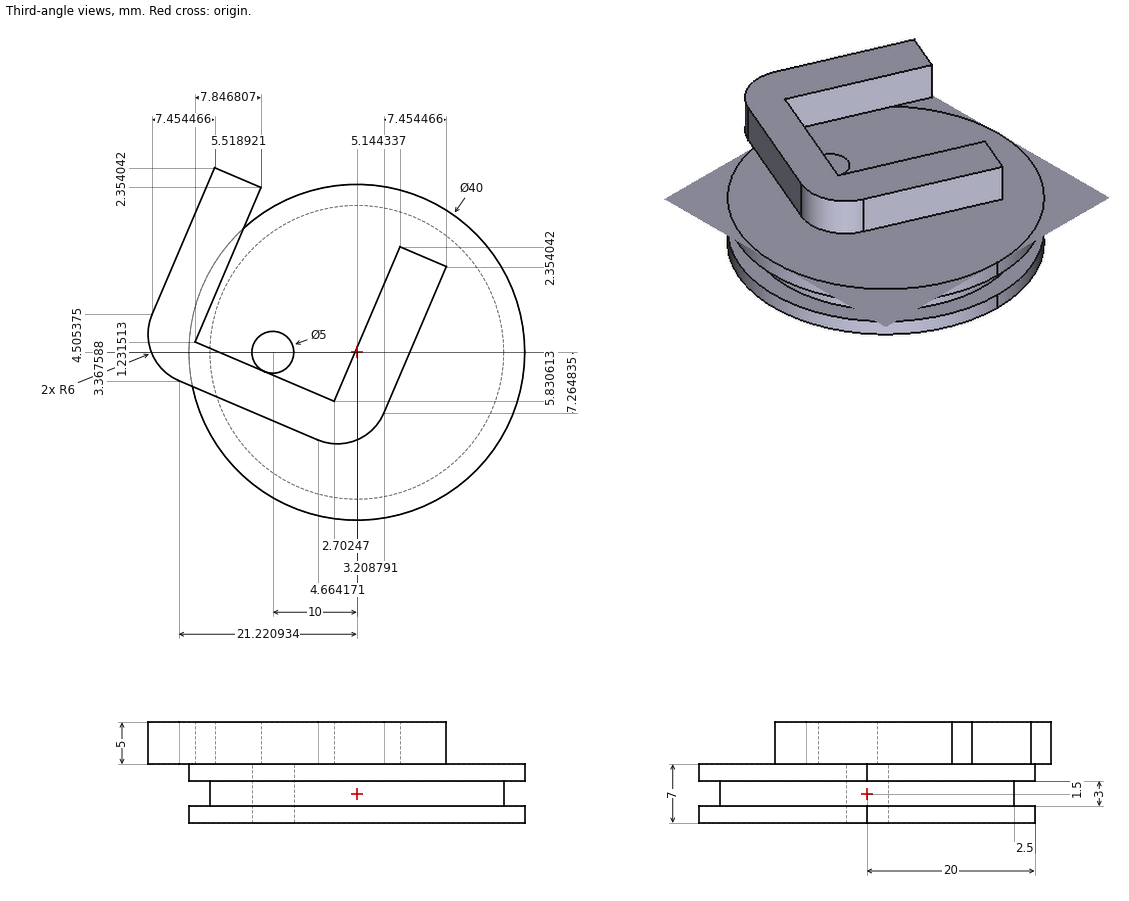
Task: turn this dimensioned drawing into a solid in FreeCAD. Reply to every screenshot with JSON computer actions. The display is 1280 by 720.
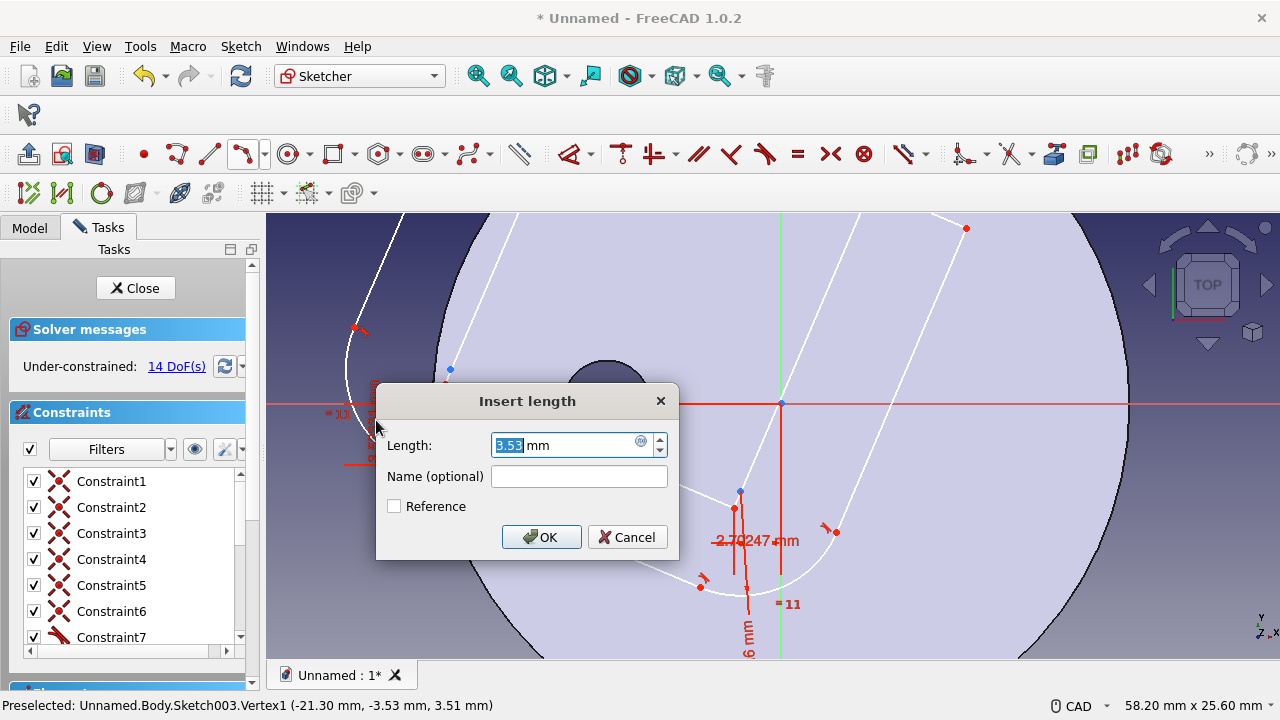
{"action": "type", "text": "3.367588"}
{"action": "key", "text": "Return"}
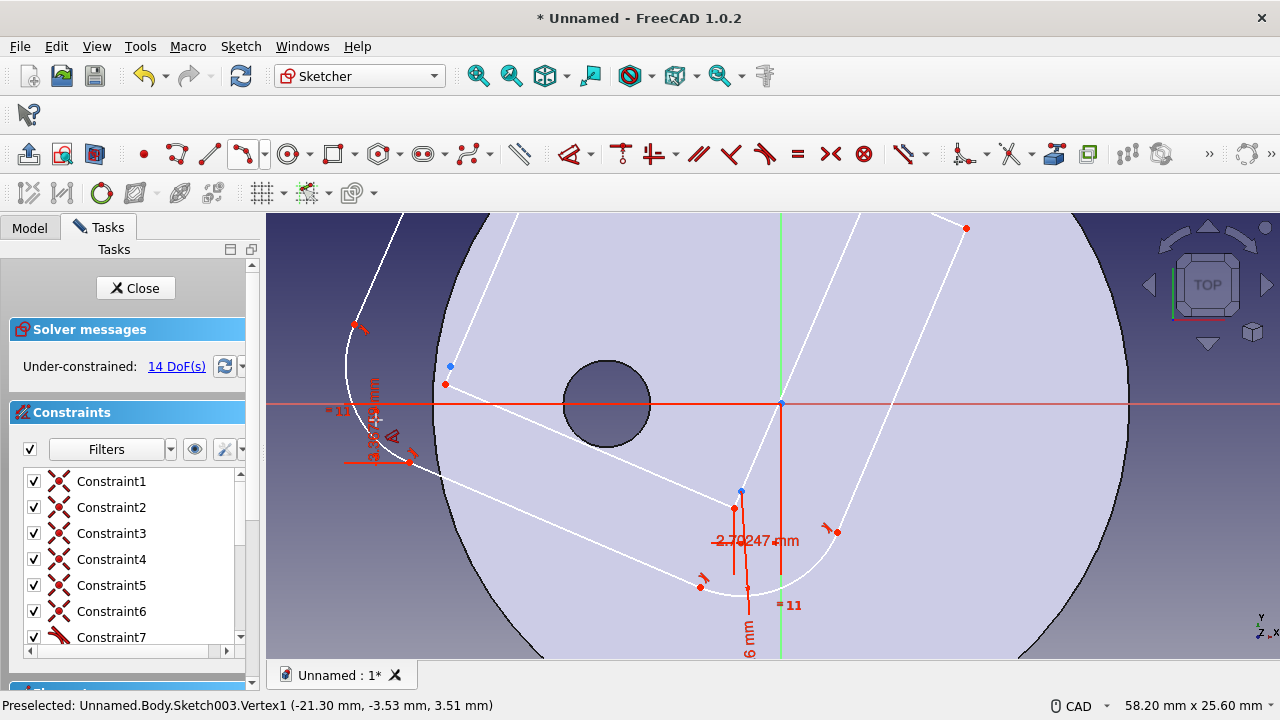
{"action": "left_click", "coordinate": [700, 588]}
{"action": "left_click", "coordinate": [741, 622]}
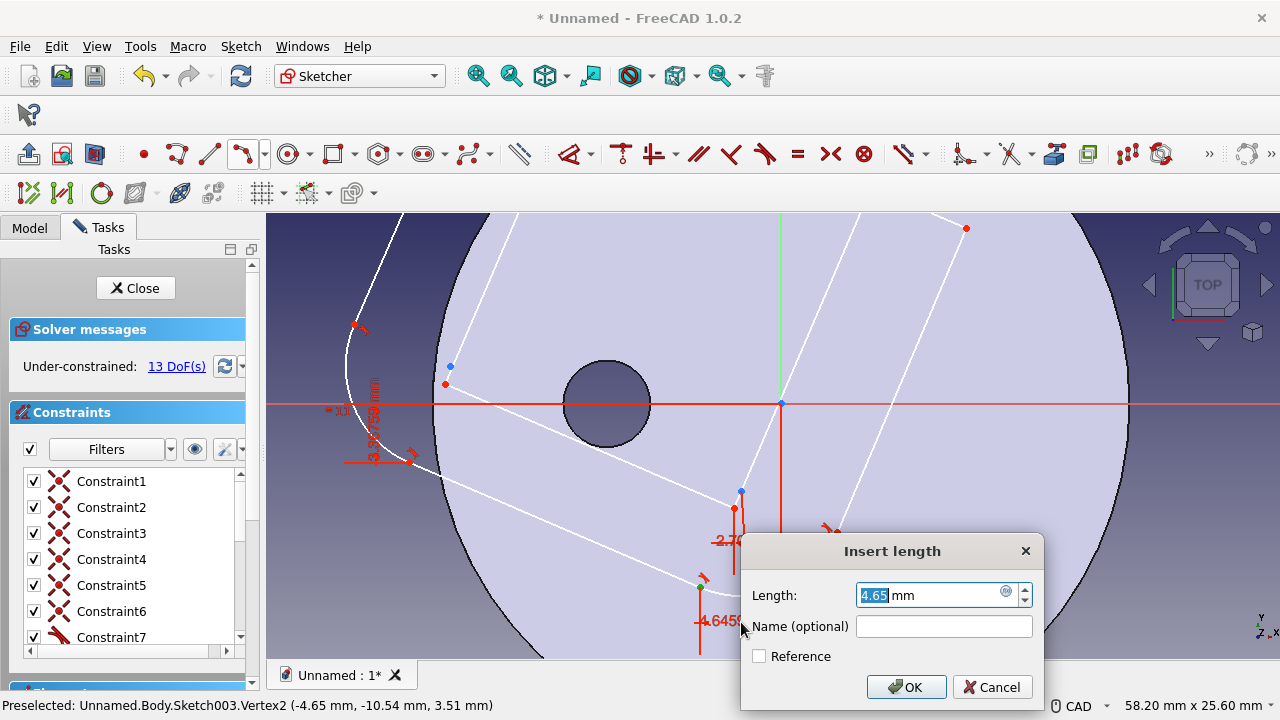
{"action": "type", "text": "4.664171"}
{"action": "key", "text": "Return"}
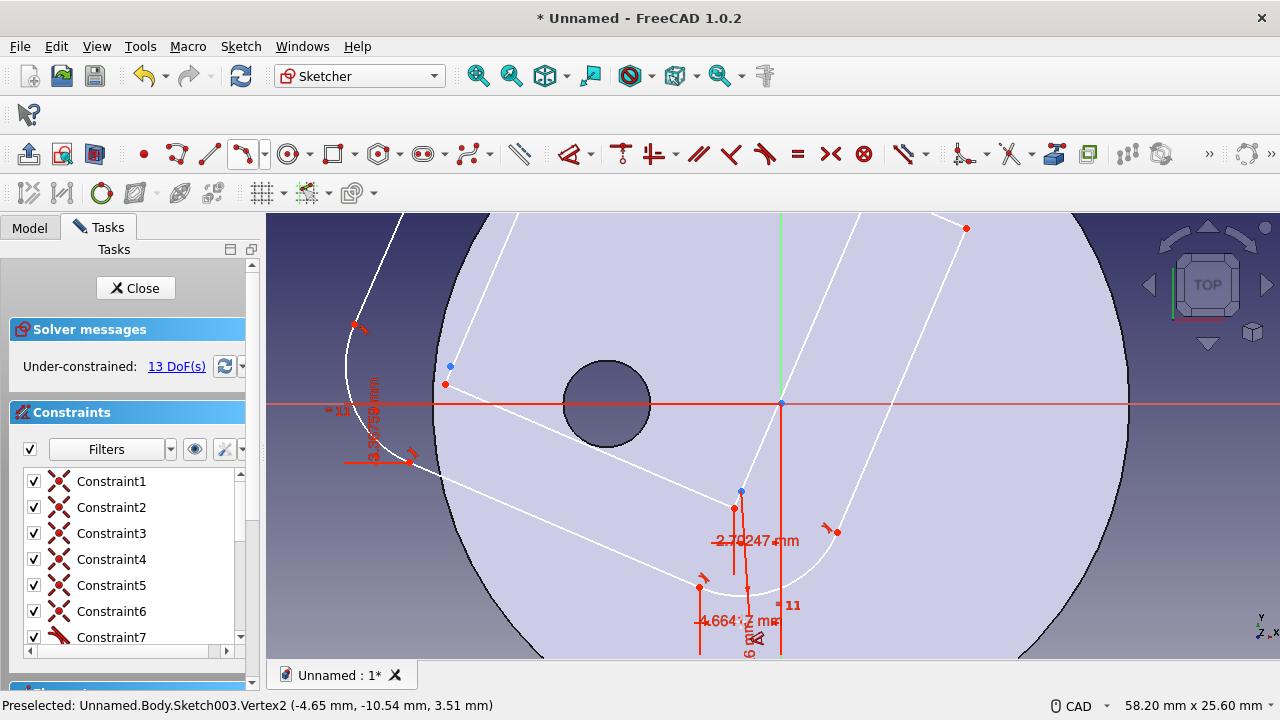
{"action": "left_click", "coordinate": [837, 532]}
{"action": "left_click", "coordinate": [809, 370]}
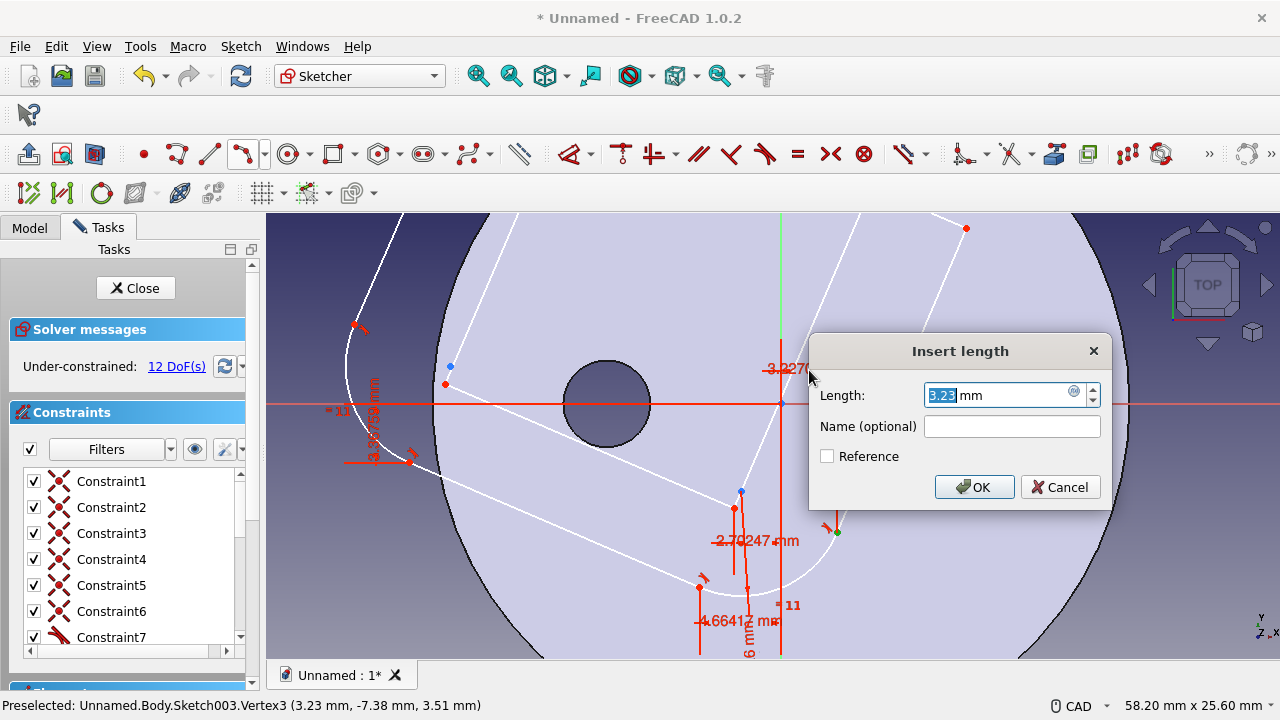
{"action": "type", "text": "3.208791"}
{"action": "key", "text": "Return"}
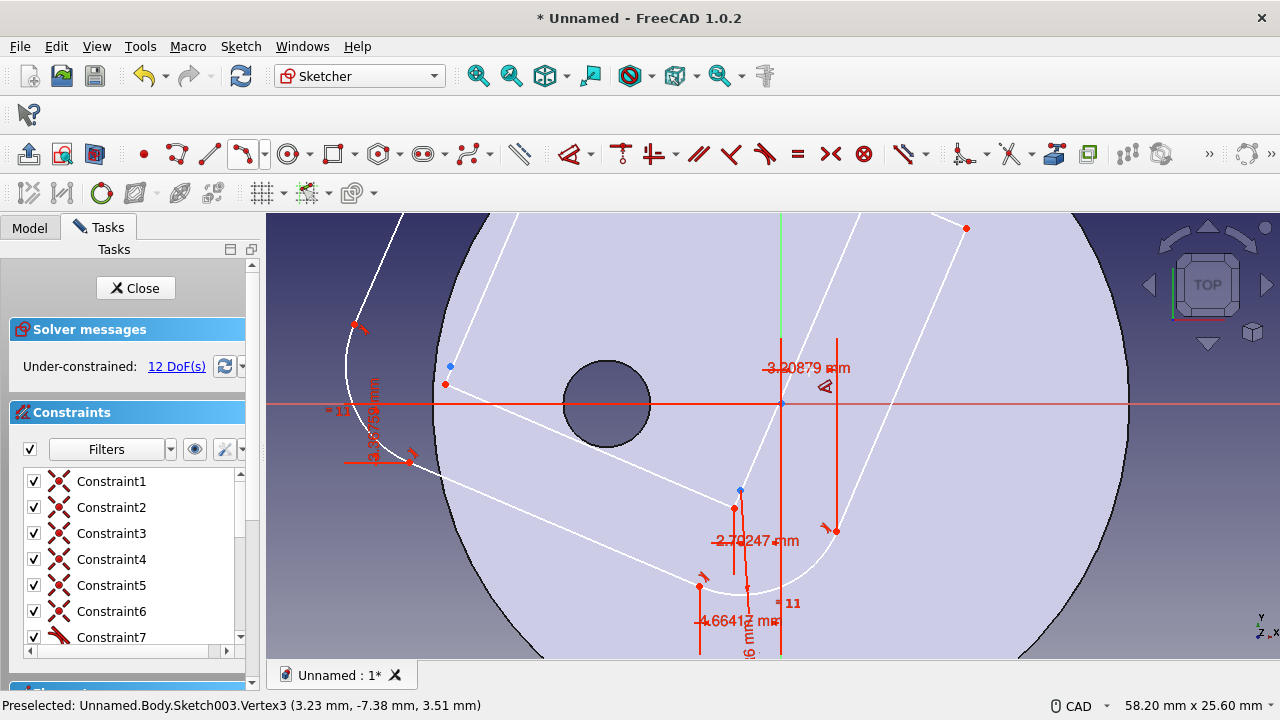
{"action": "left_click", "coordinate": [837, 531]}
{"action": "left_click", "coordinate": [871, 497]}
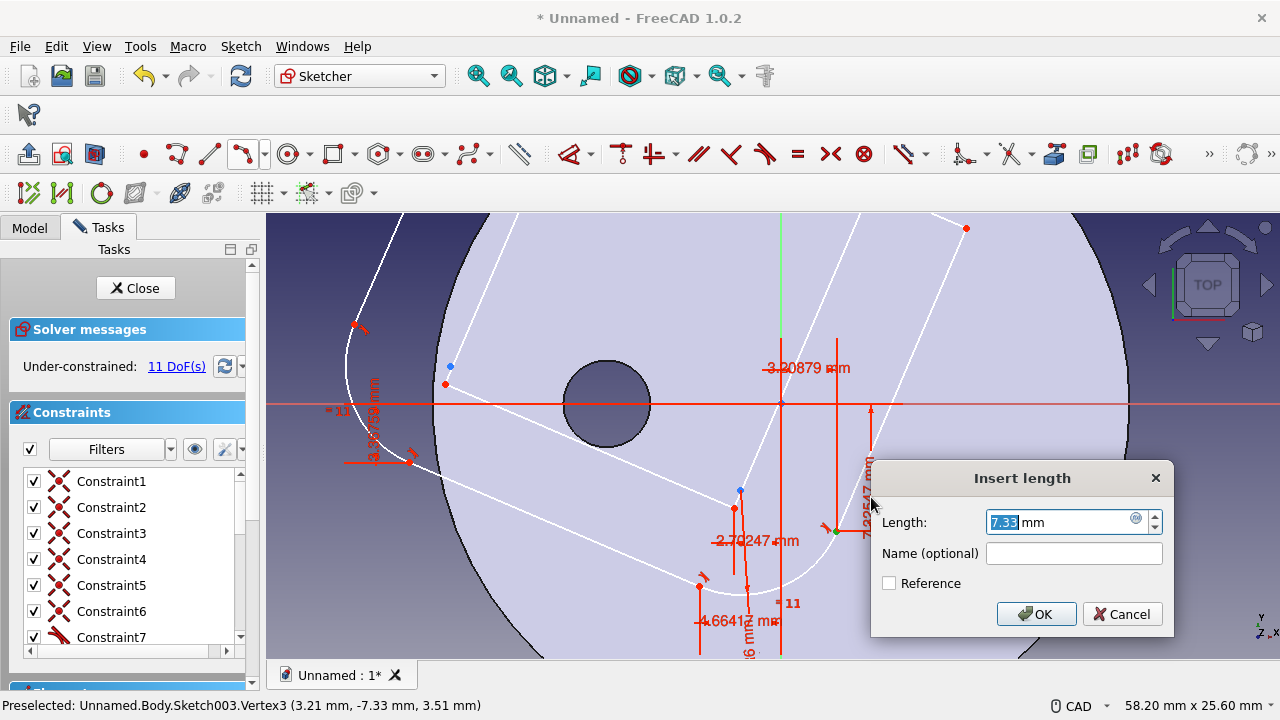
{"action": "type", "text": "7.264835"}
{"action": "key", "text": "Return"}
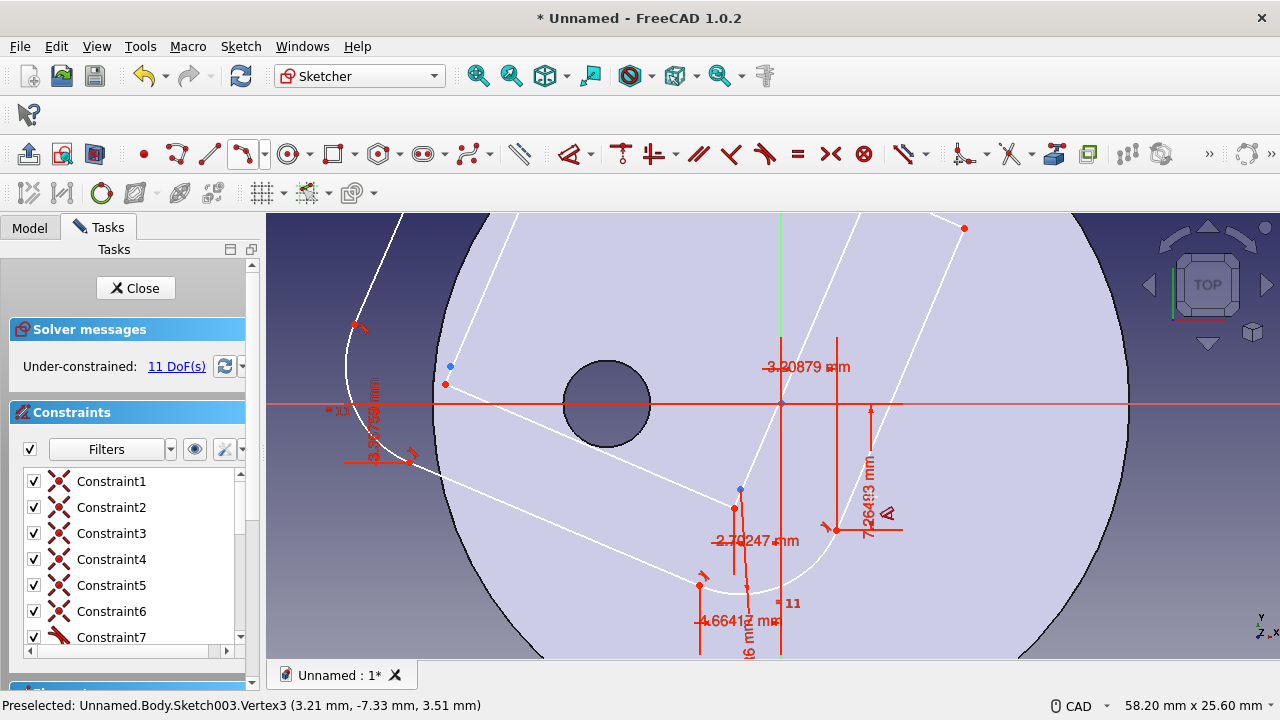
{"action": "scroll", "coordinate": [740, 544], "scroll_direction": "down", "scroll_amount": 4}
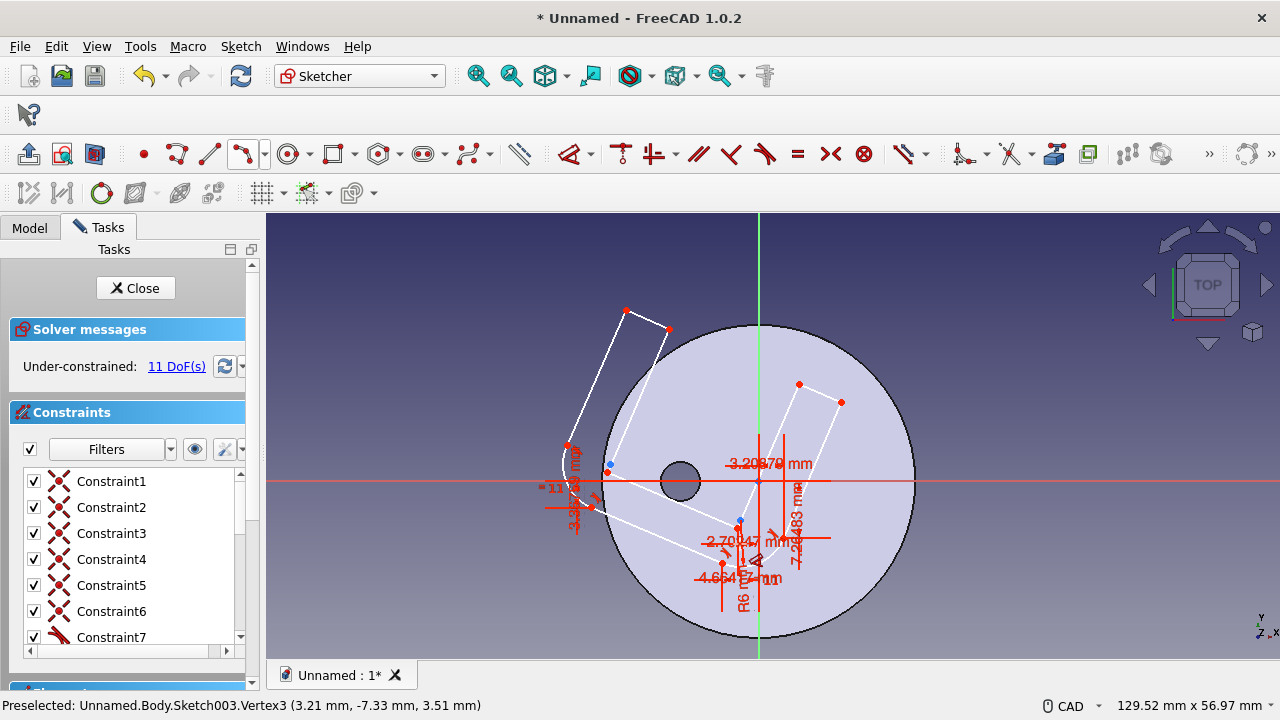
{"action": "left_click", "coordinate": [799, 384]}
{"action": "left_click", "coordinate": [779, 350]}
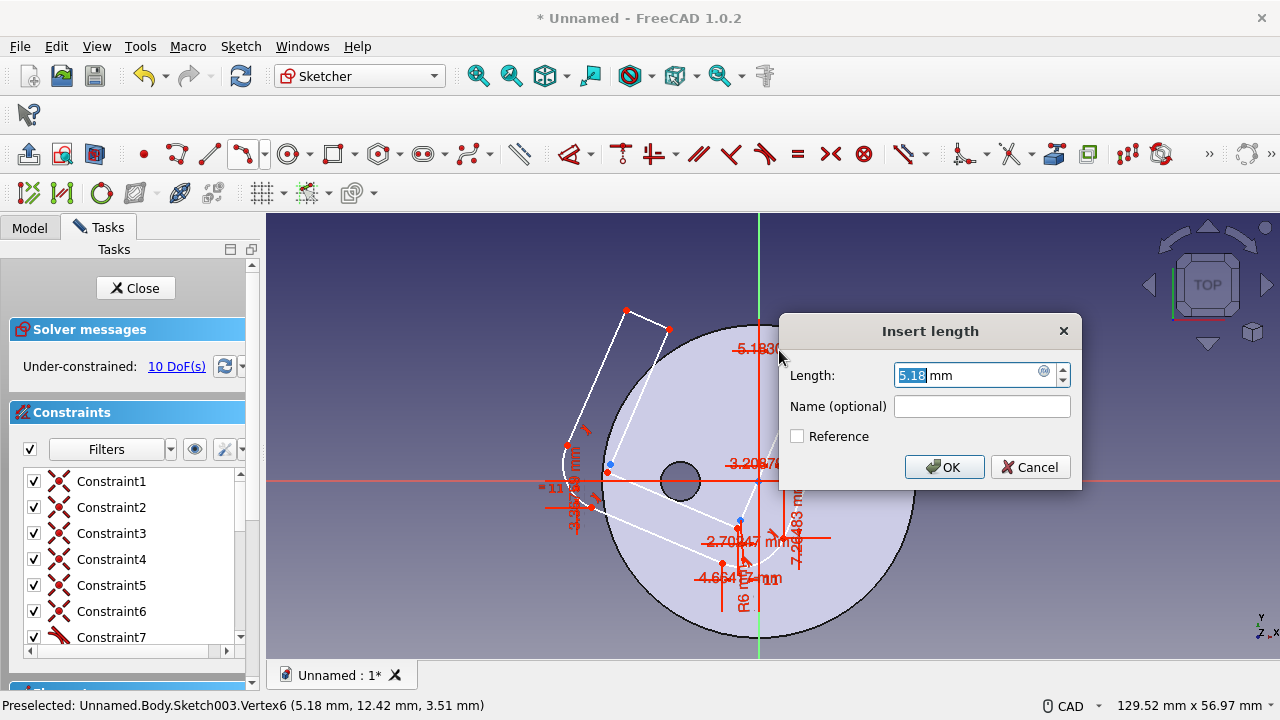
{"action": "type", "text": "5.144337"}
{"action": "key", "text": "Return"}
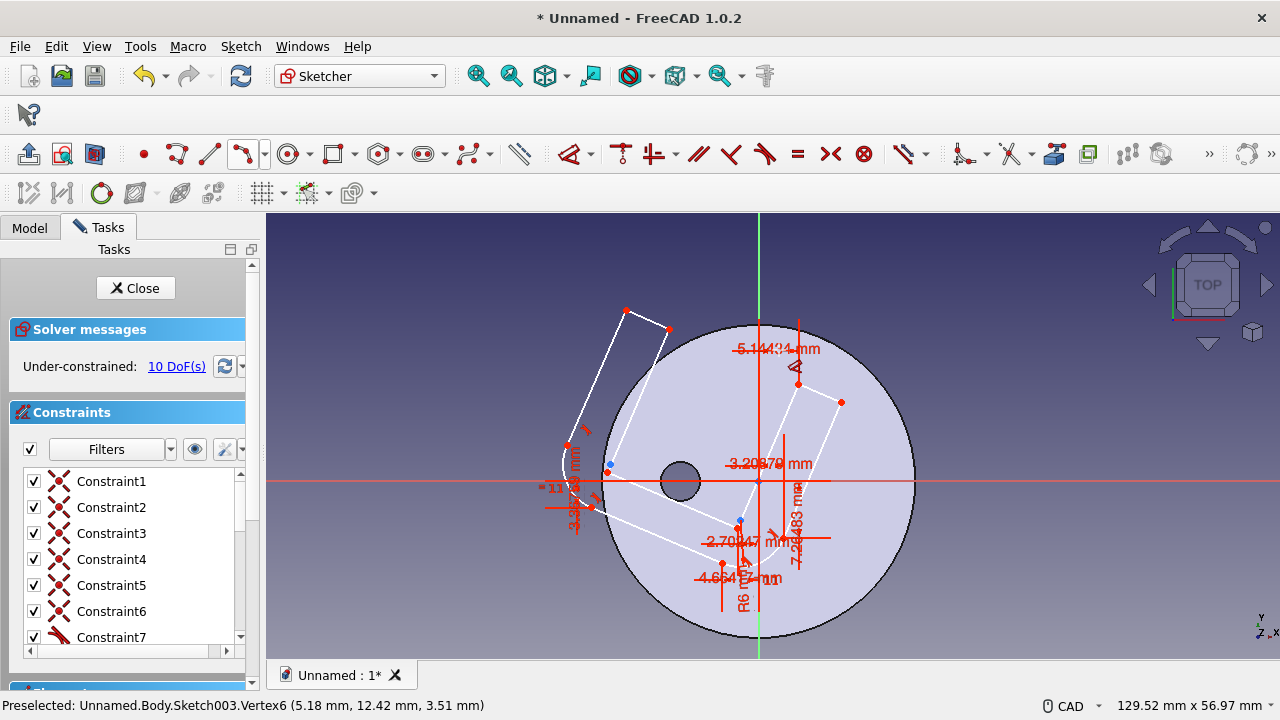
{"action": "scroll", "coordinate": [738, 528], "scroll_direction": "up", "scroll_amount": 2}